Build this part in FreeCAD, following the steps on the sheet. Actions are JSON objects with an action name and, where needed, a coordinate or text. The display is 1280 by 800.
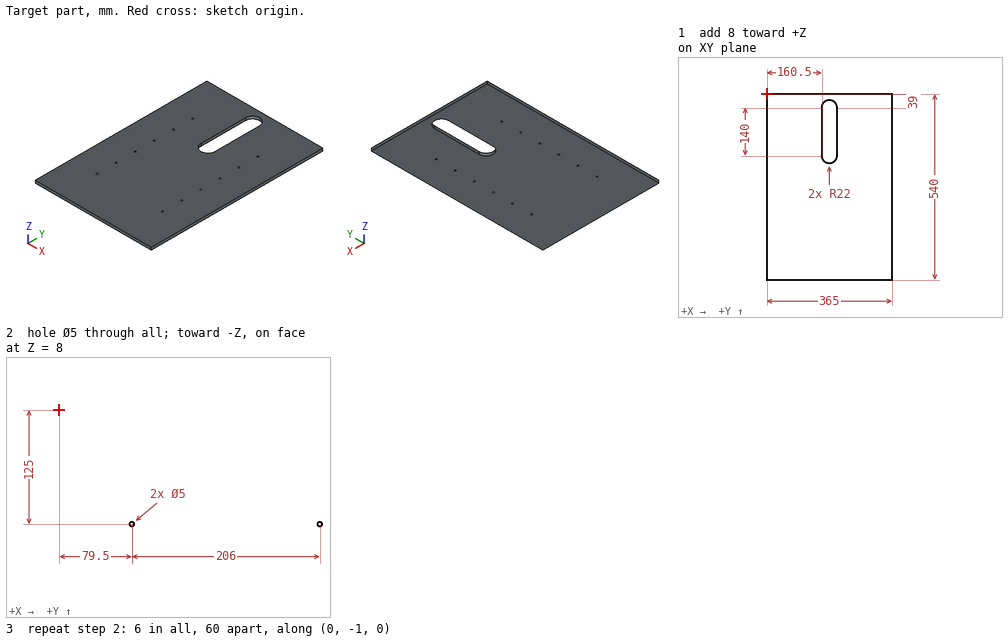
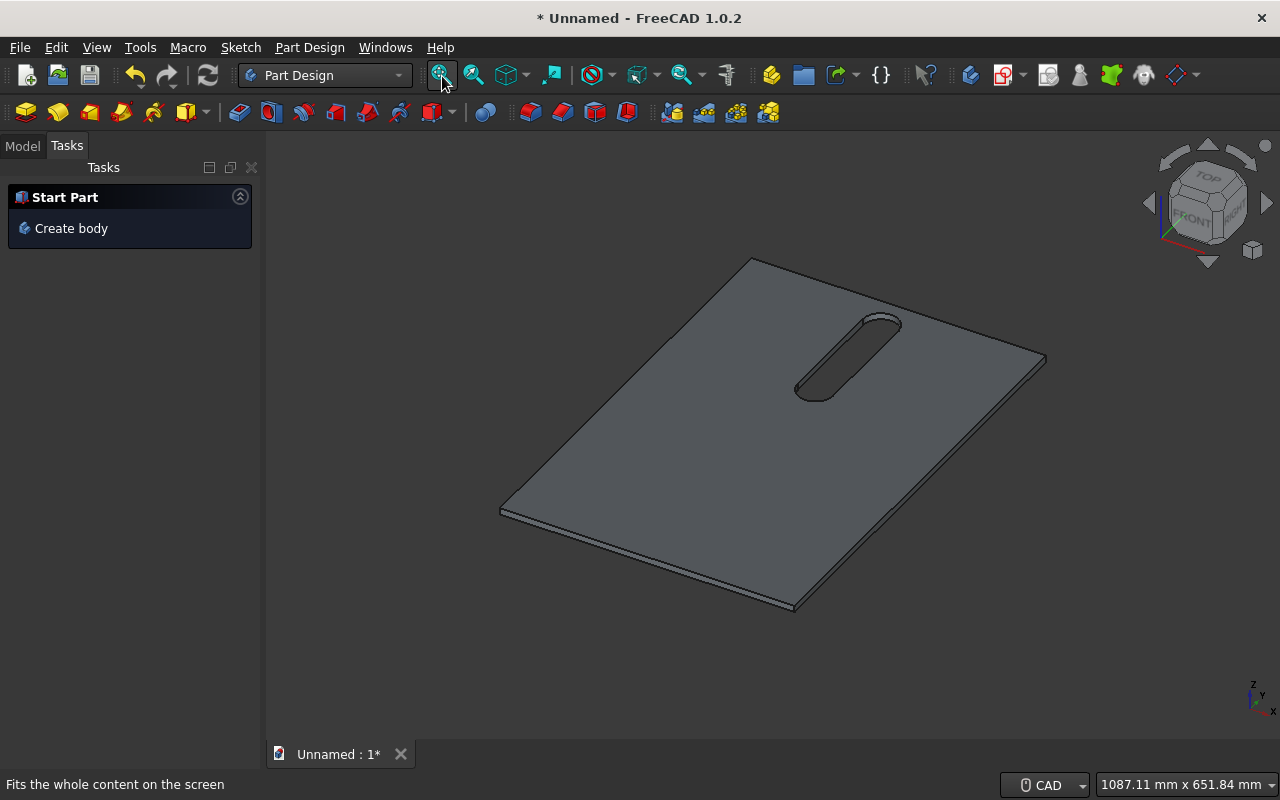
{"action": "left_click", "coordinate": [737, 467]}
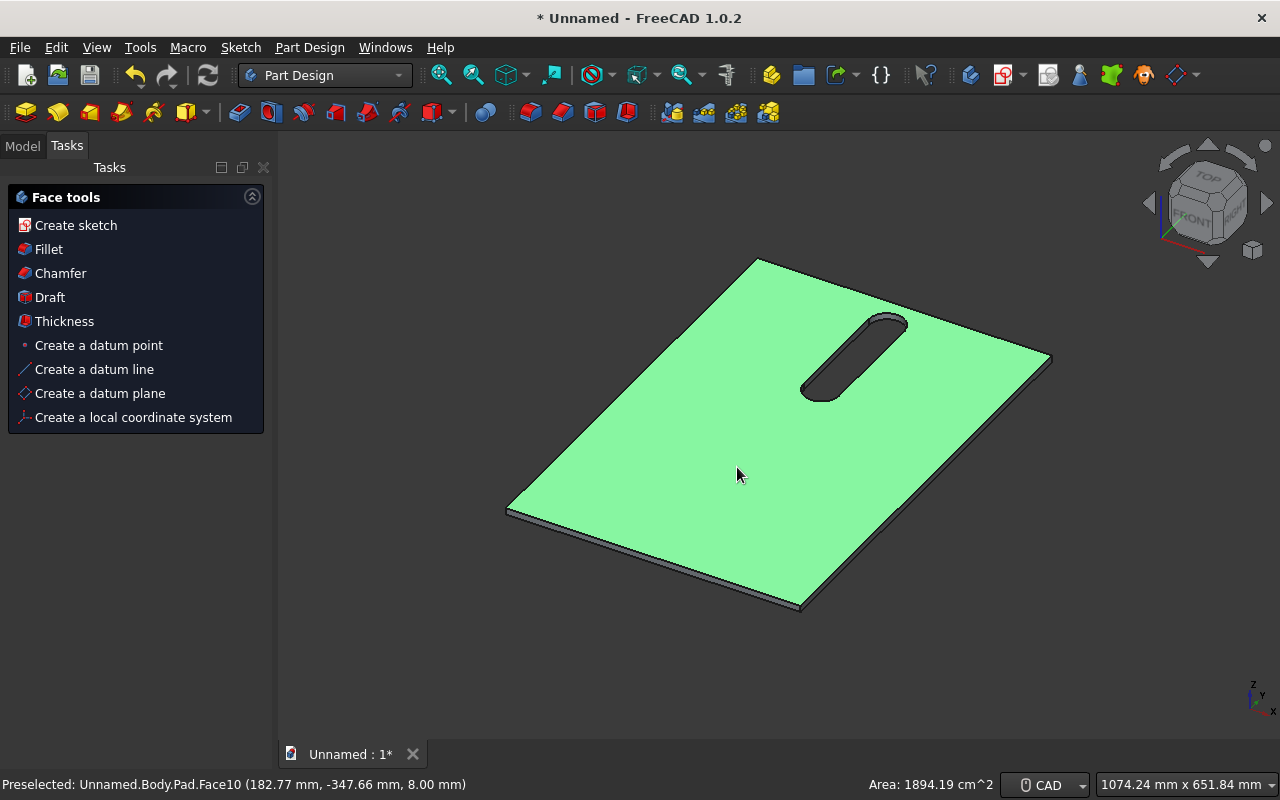
{"action": "left_click", "coordinate": [1004, 76]}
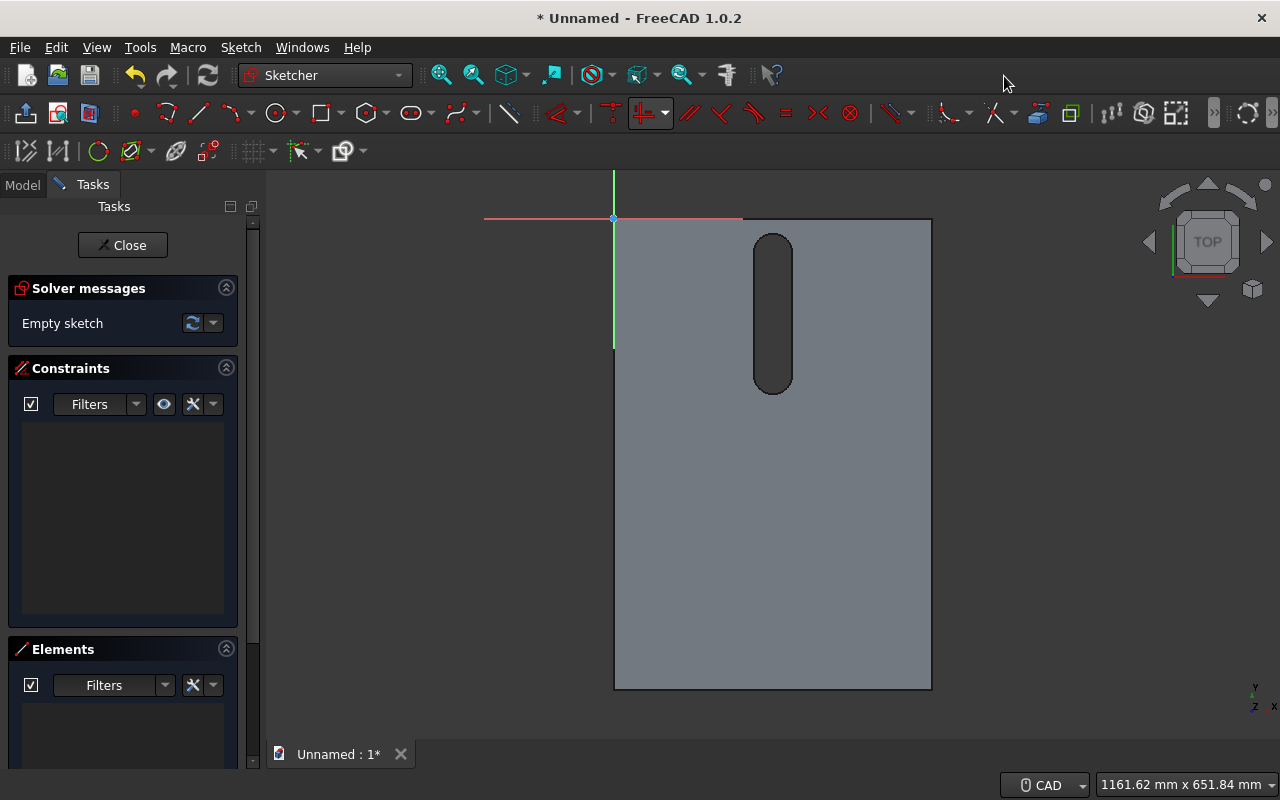
{"action": "scroll", "coordinate": [768, 198], "scroll_direction": "up", "scroll_amount": 4}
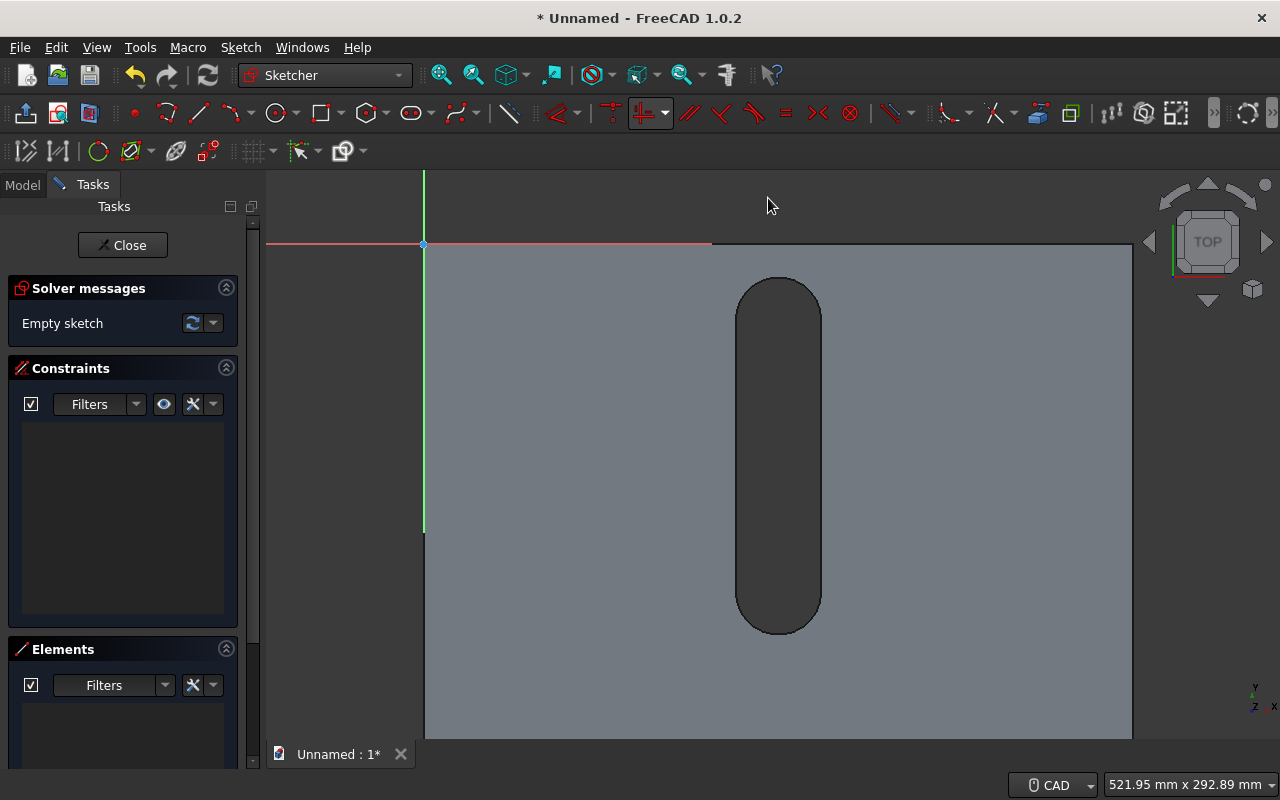
{"action": "left_click", "coordinate": [276, 114]}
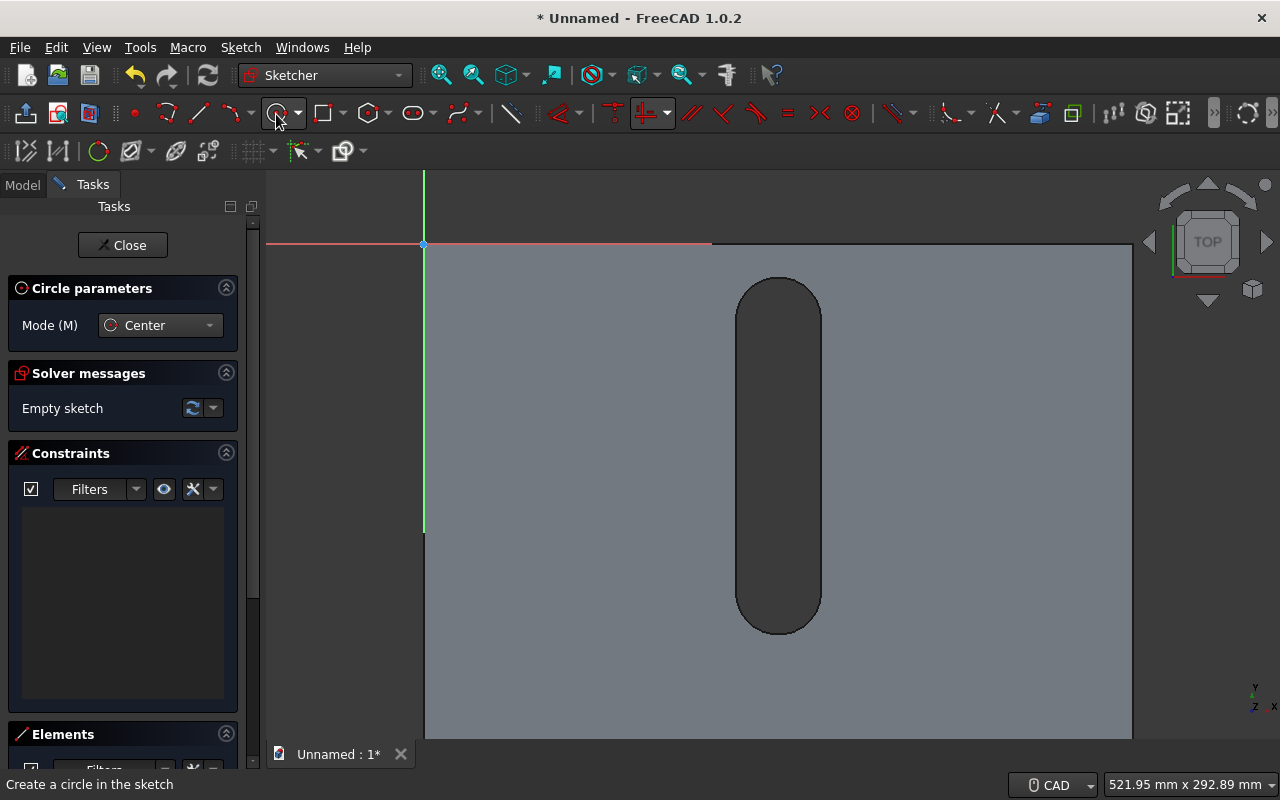
{"action": "scroll", "coordinate": [578, 487], "scroll_direction": "up", "scroll_amount": 8}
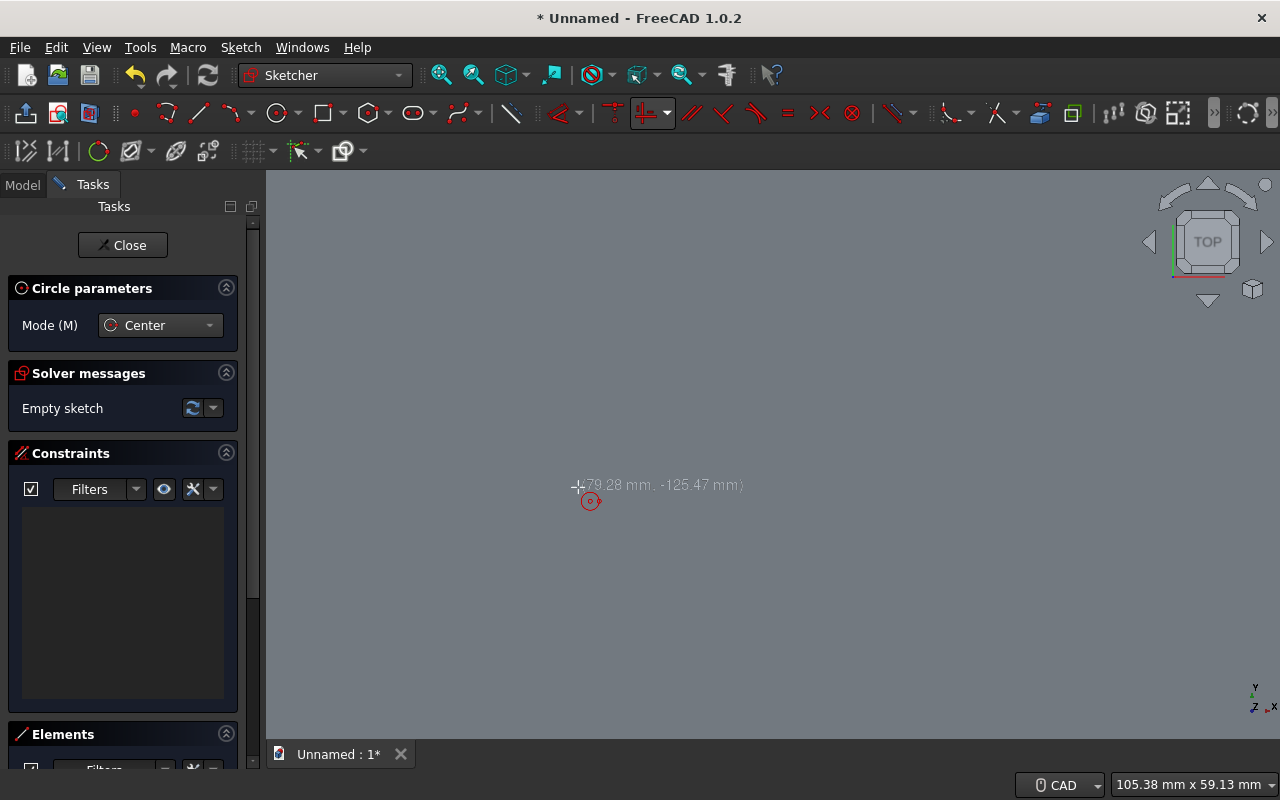
{"action": "scroll", "coordinate": [579, 596], "scroll_direction": "down", "scroll_amount": 8}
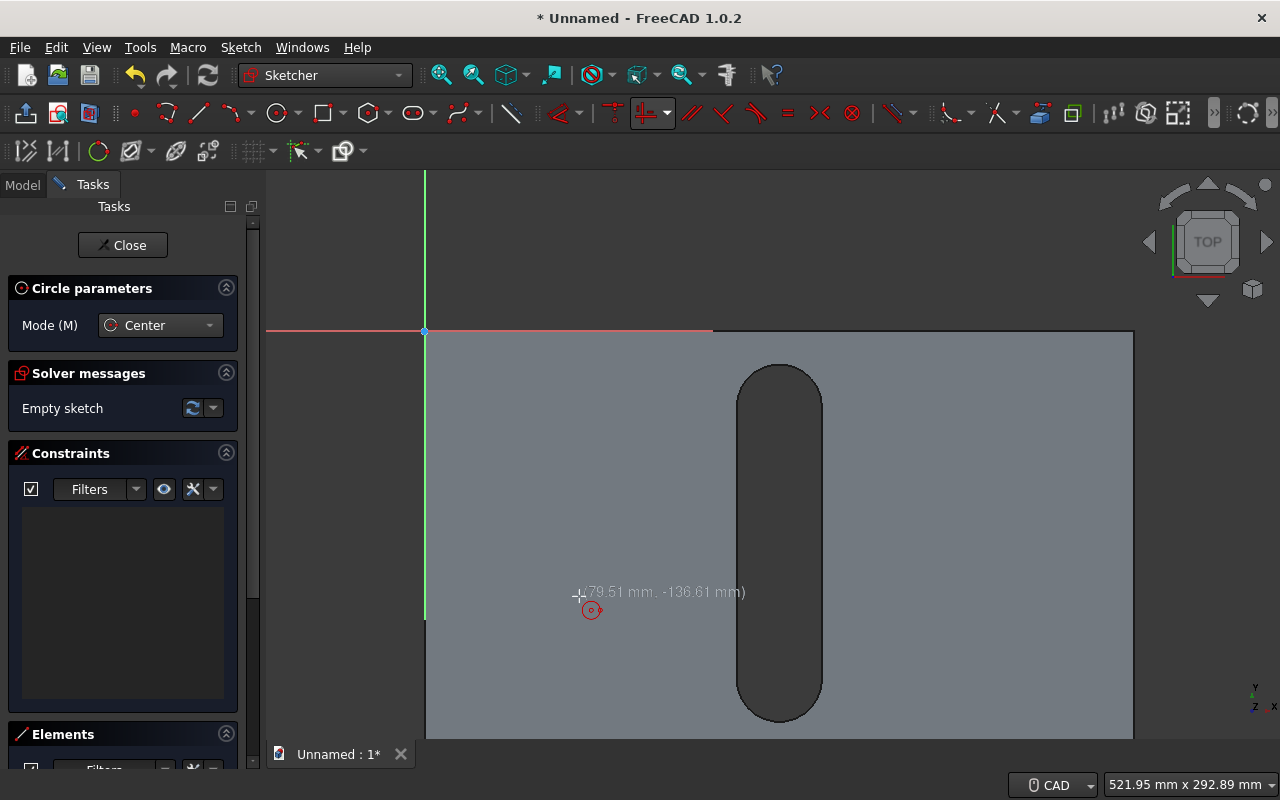
{"action": "left_click", "coordinate": [579, 574]}
{"action": "mouse_move", "coordinate": [583, 571]}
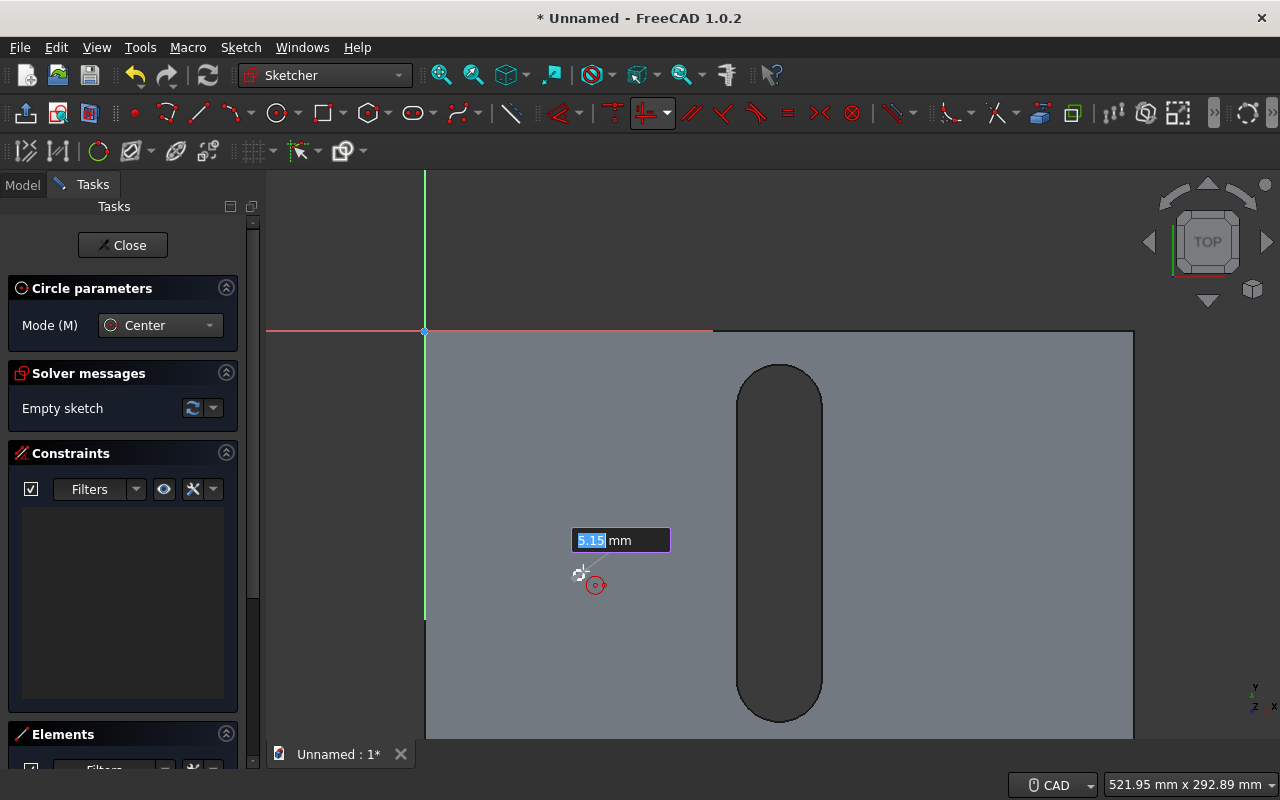
{"action": "type", "text": "5"}
{"action": "key", "text": "Return"}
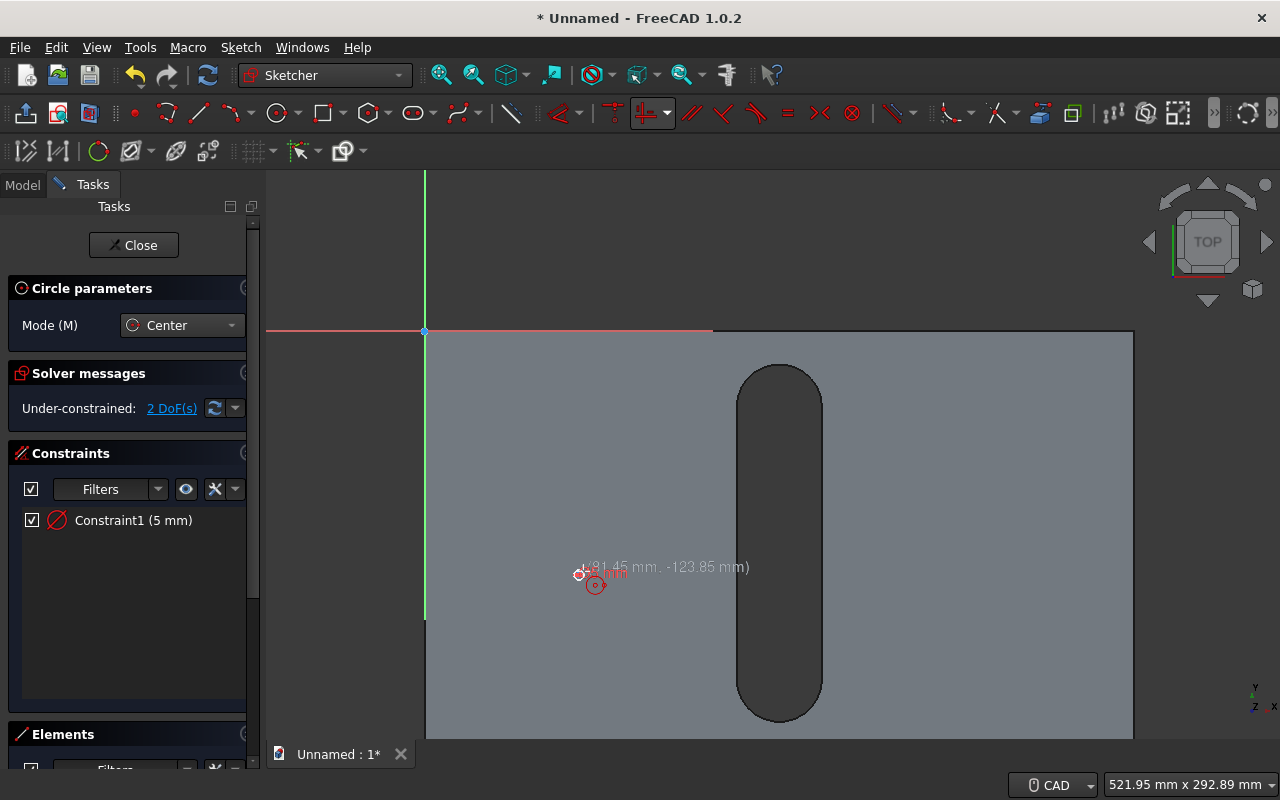
{"action": "scroll", "coordinate": [979, 574], "scroll_direction": "up", "scroll_amount": 8}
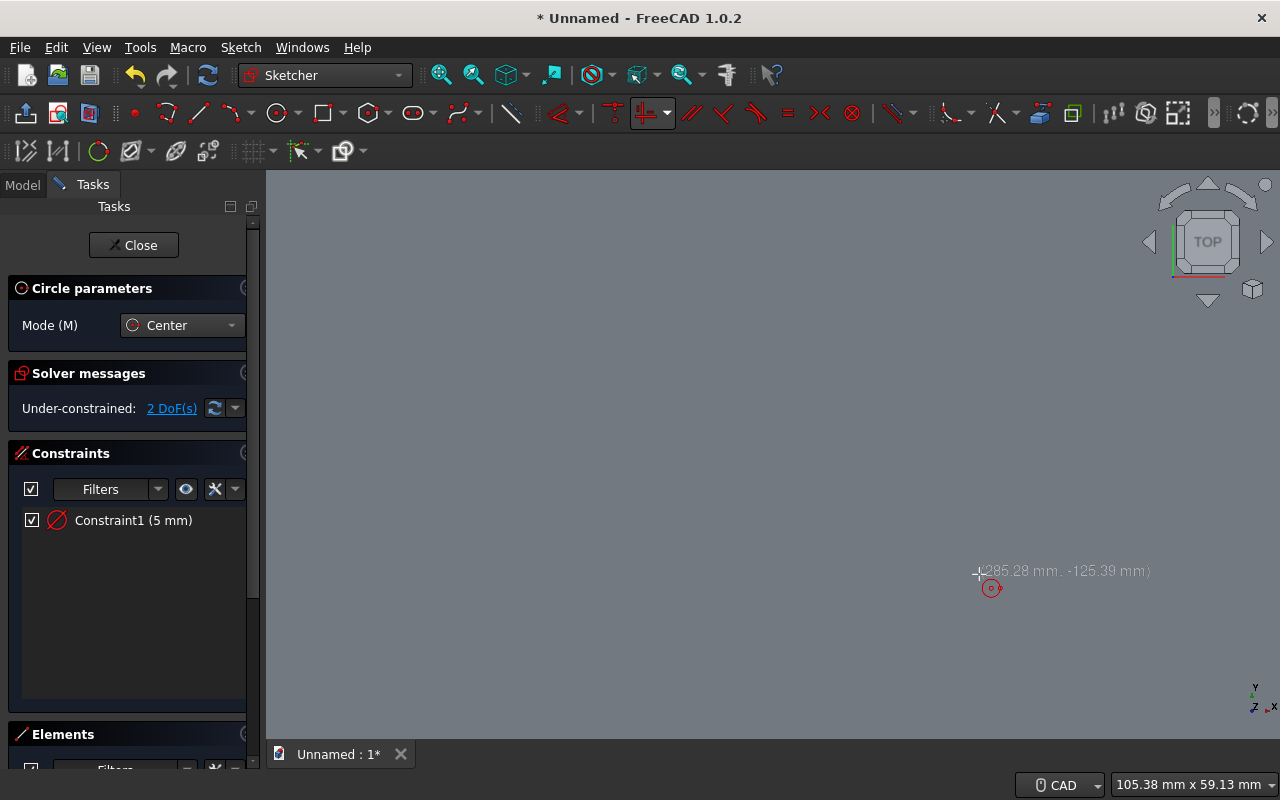
{"action": "scroll", "coordinate": [980, 574], "scroll_direction": "down", "scroll_amount": 8}